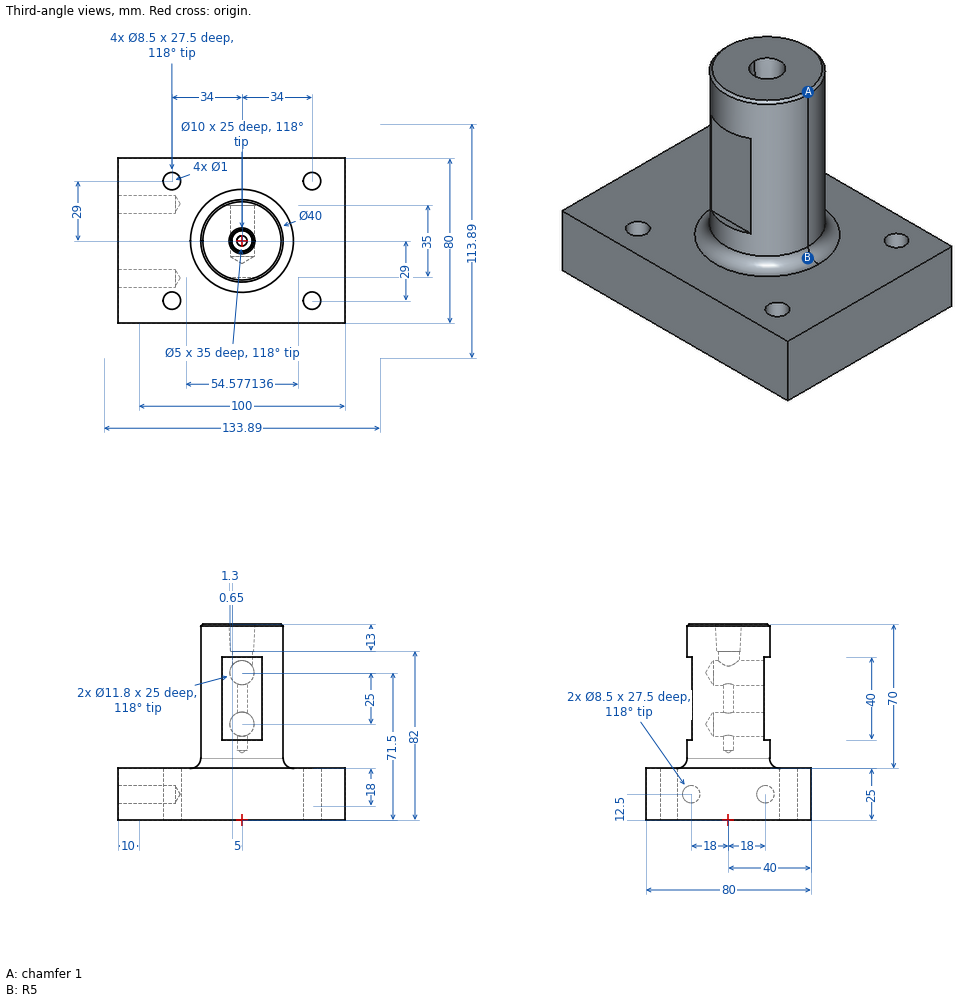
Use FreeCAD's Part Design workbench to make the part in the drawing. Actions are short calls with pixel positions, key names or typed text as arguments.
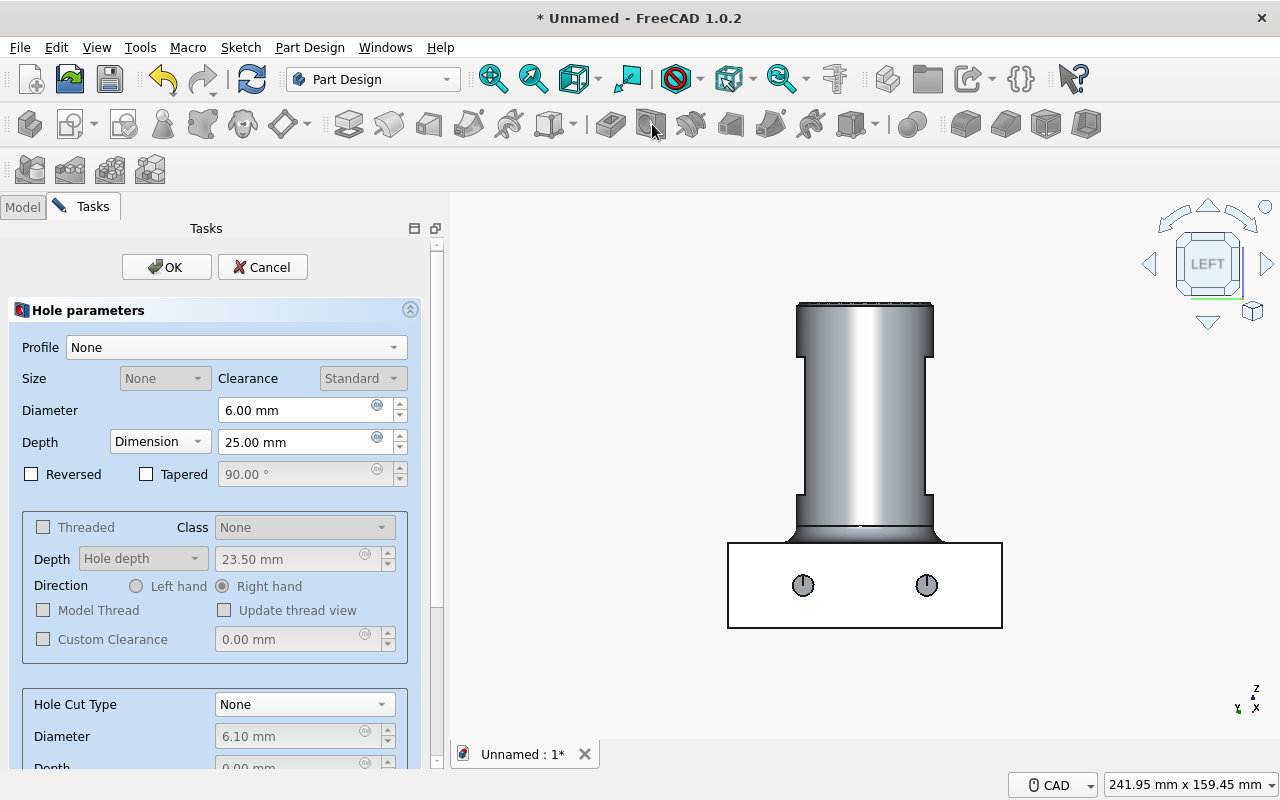
triple_click(305, 410)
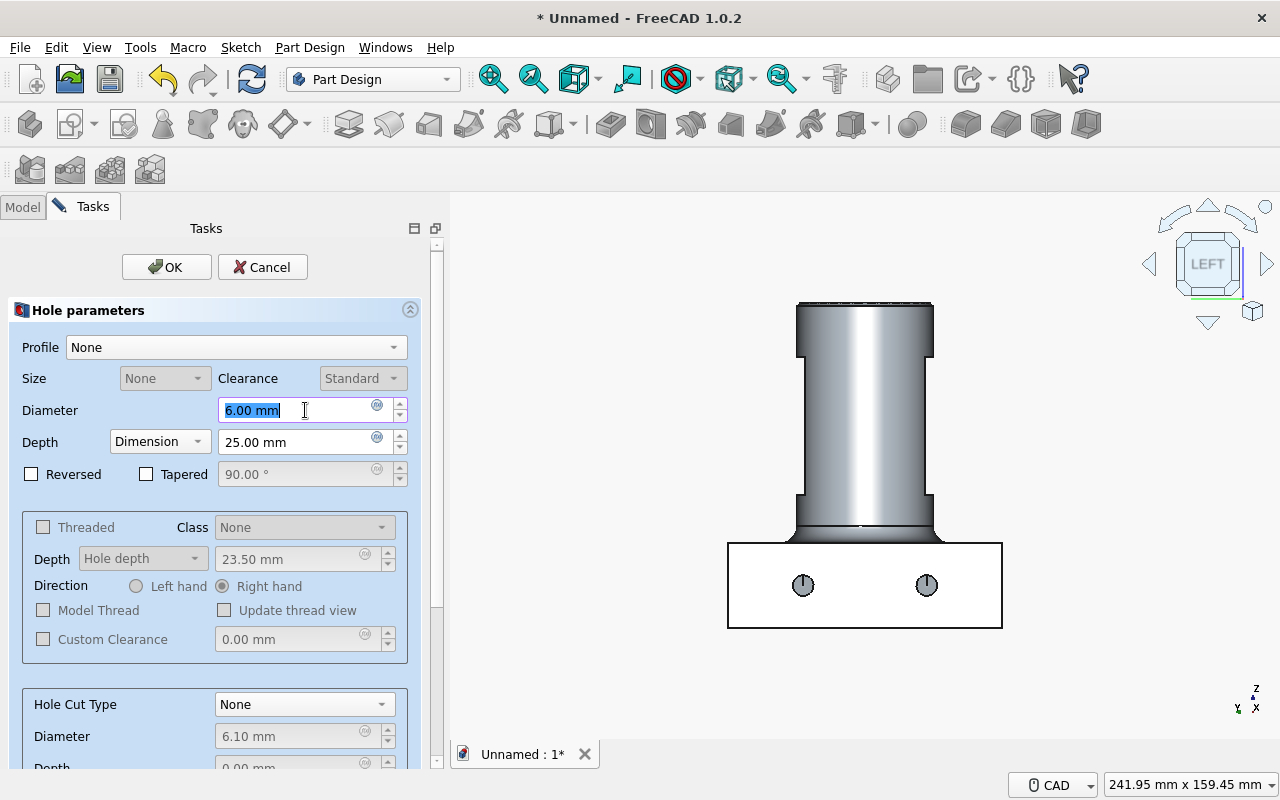
text(8.5)
key(Tab)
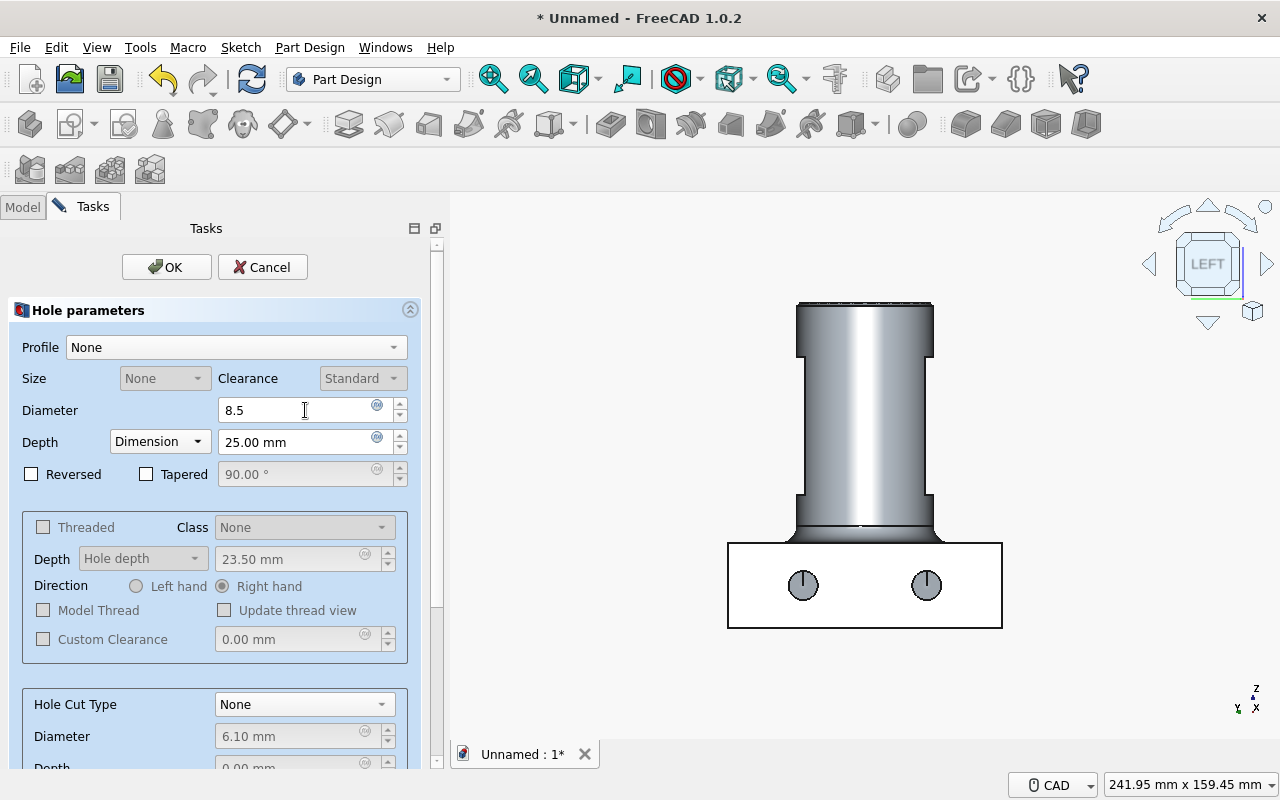
triple_click(305, 442)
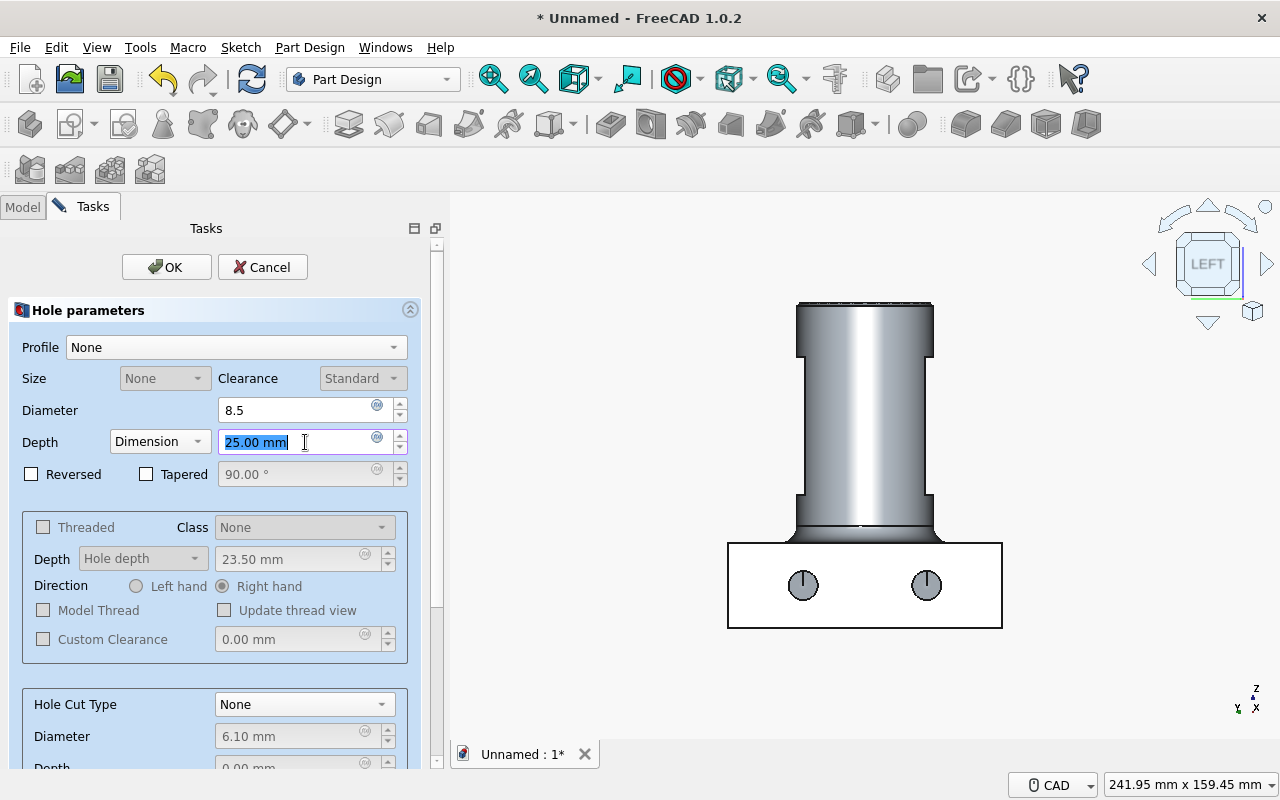
text(27.5)
key(Tab)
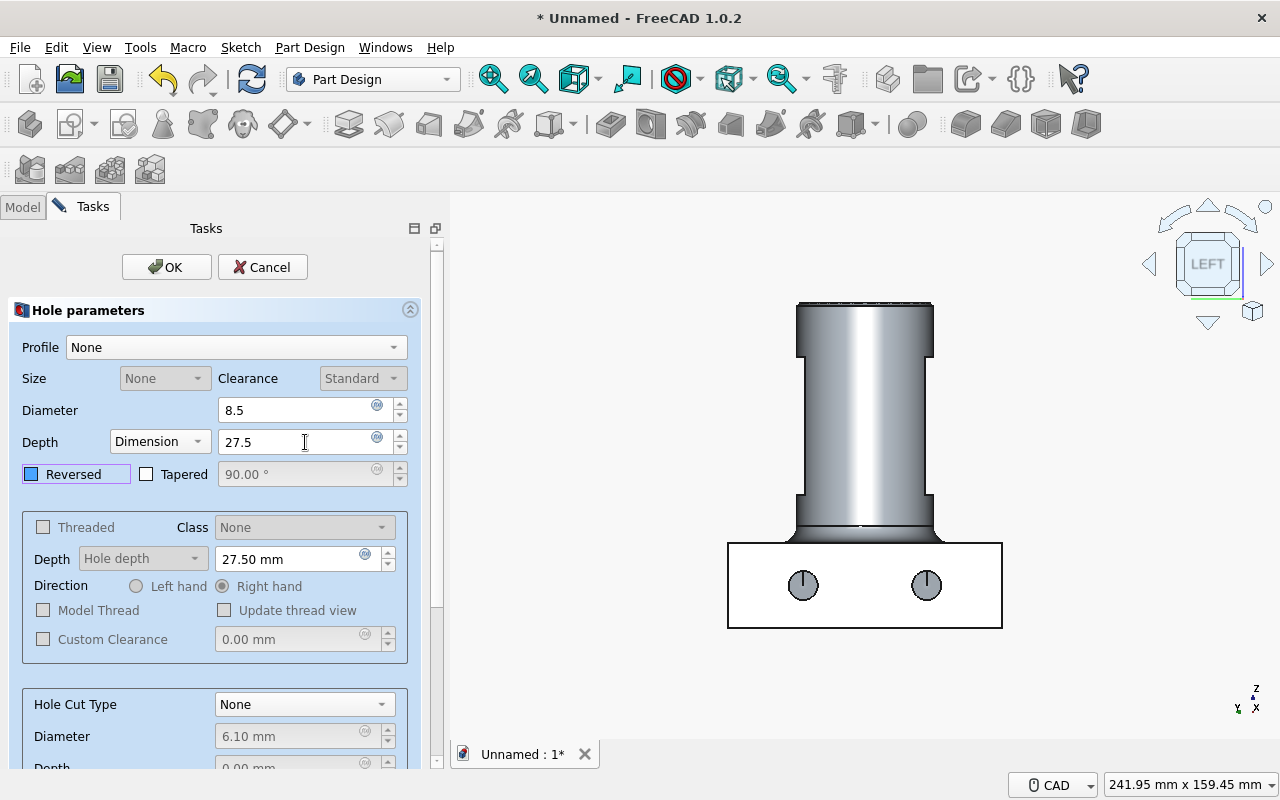
click(167, 267)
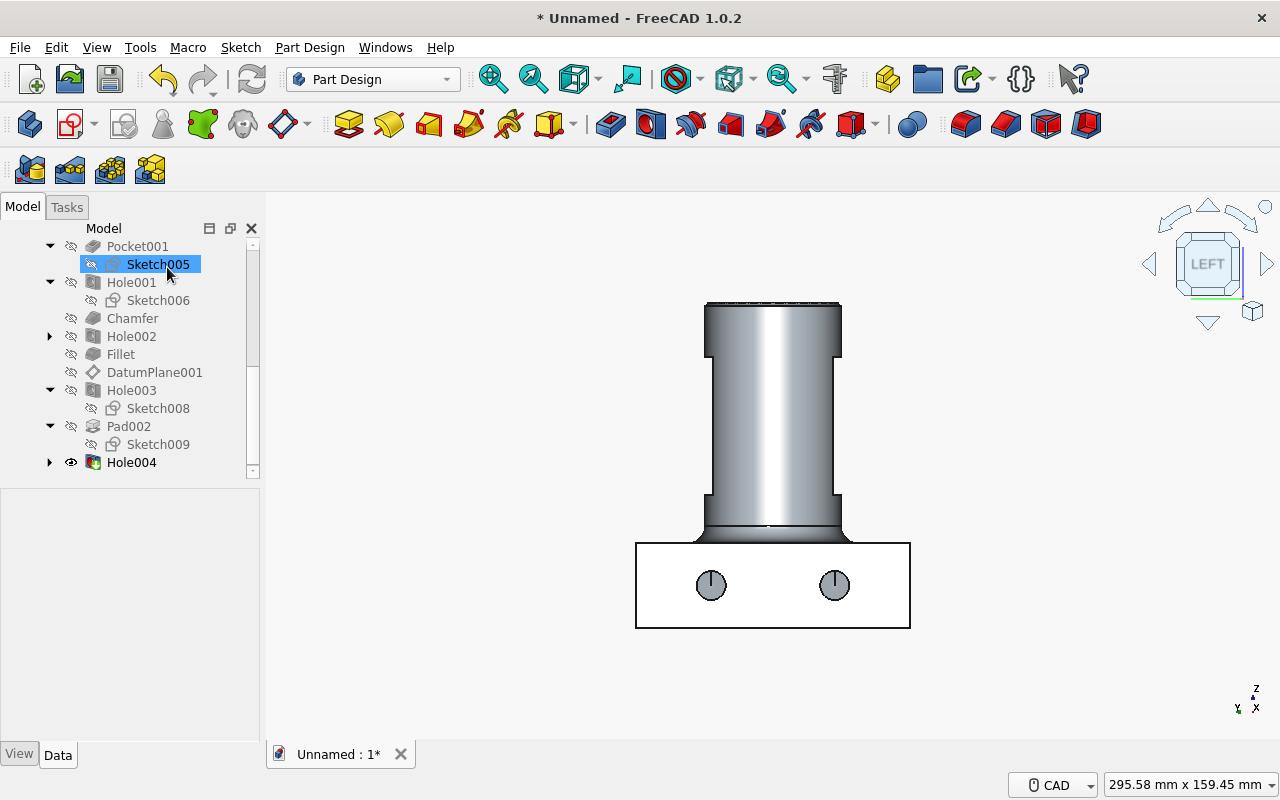
key(0)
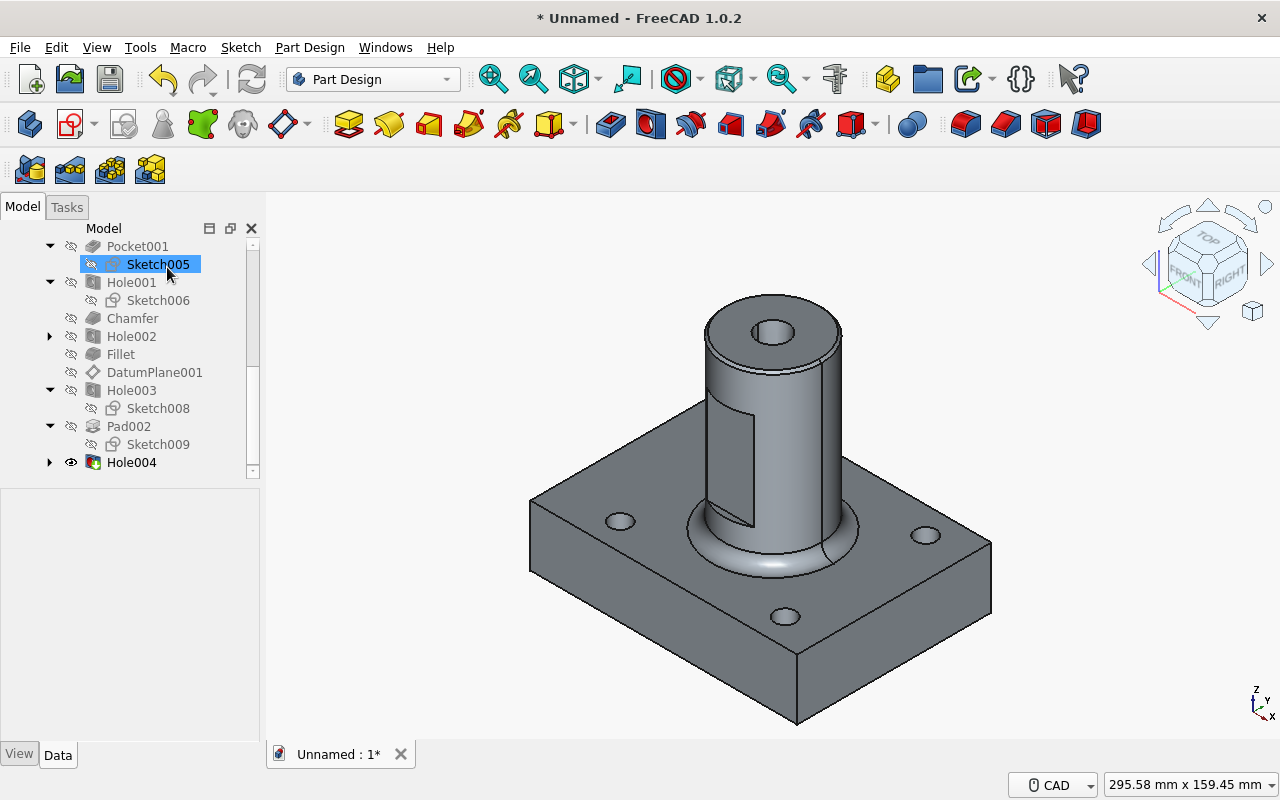
key(v)
key(f)